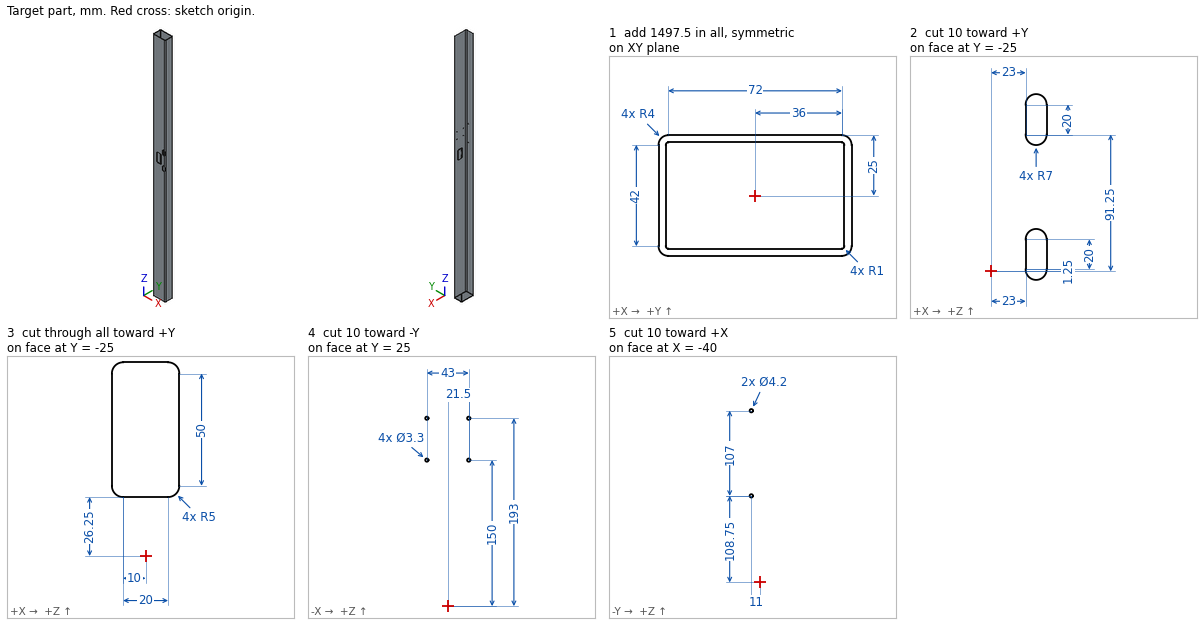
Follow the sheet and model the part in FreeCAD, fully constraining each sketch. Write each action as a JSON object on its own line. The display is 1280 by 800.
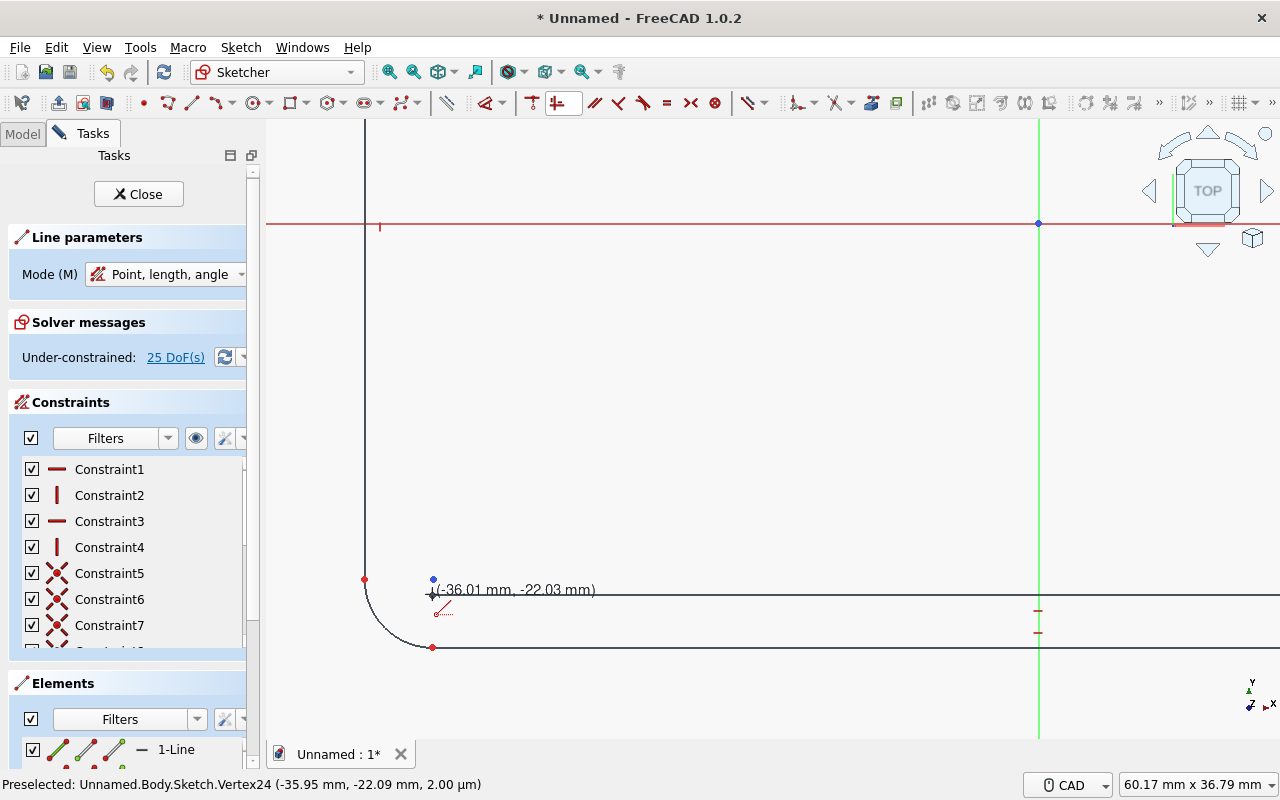
{"action": "left_click", "coordinate": [415, 578]}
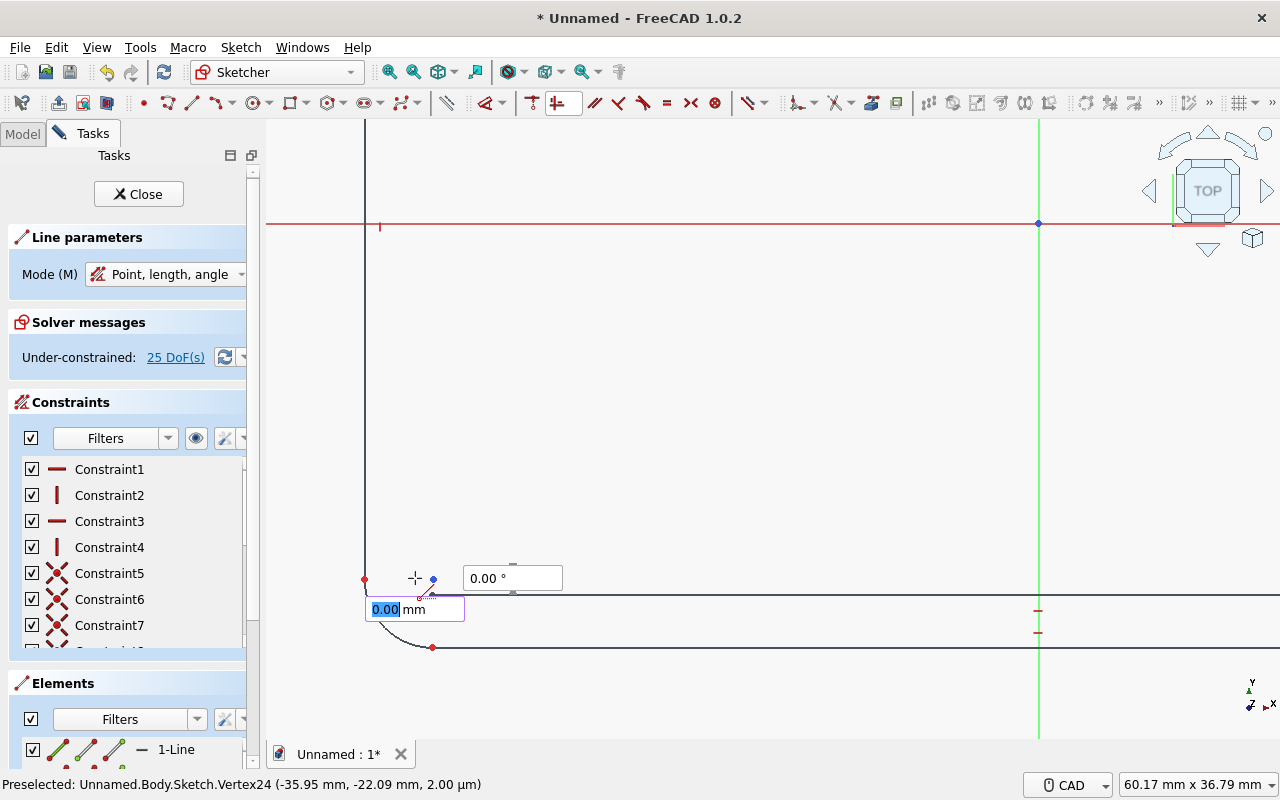
{"action": "scroll", "coordinate": [432, 596], "scroll_direction": "down", "scroll_amount": 4}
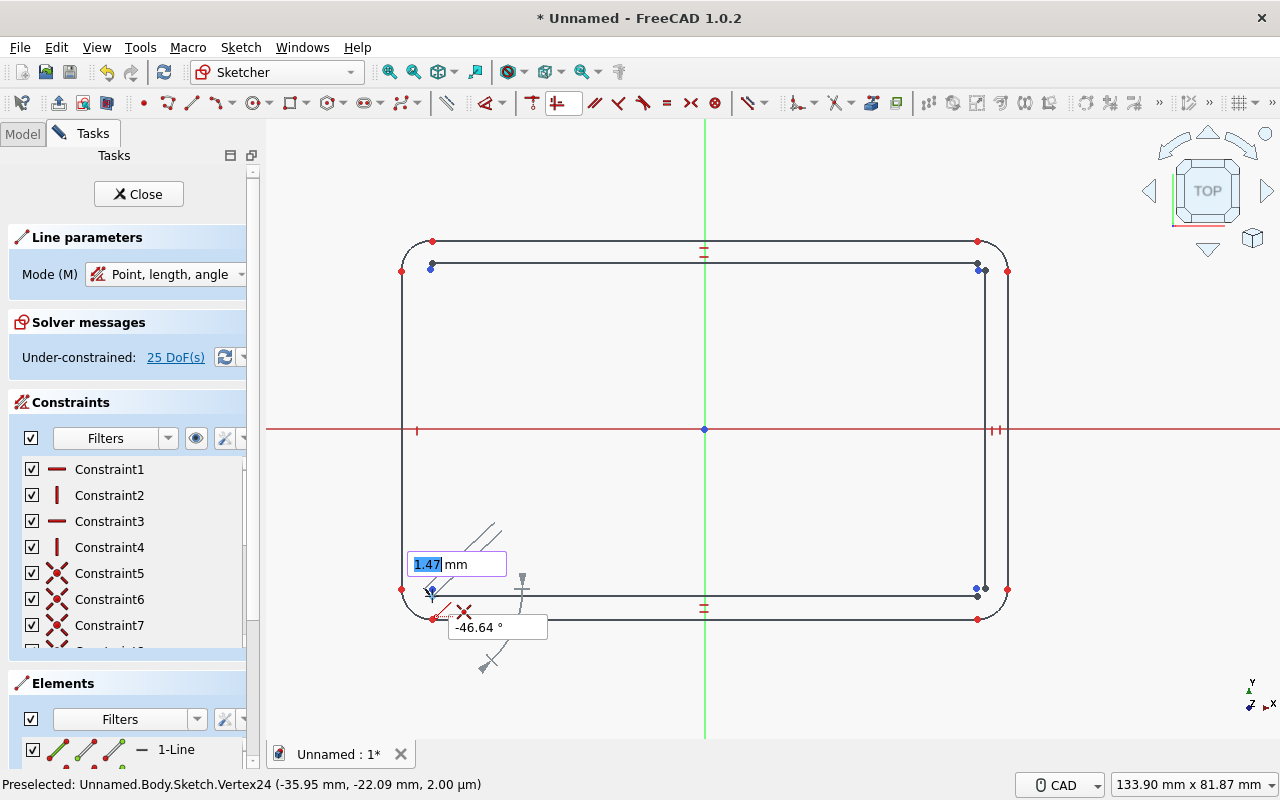
{"action": "scroll", "coordinate": [425, 270], "scroll_direction": "up", "scroll_amount": 4}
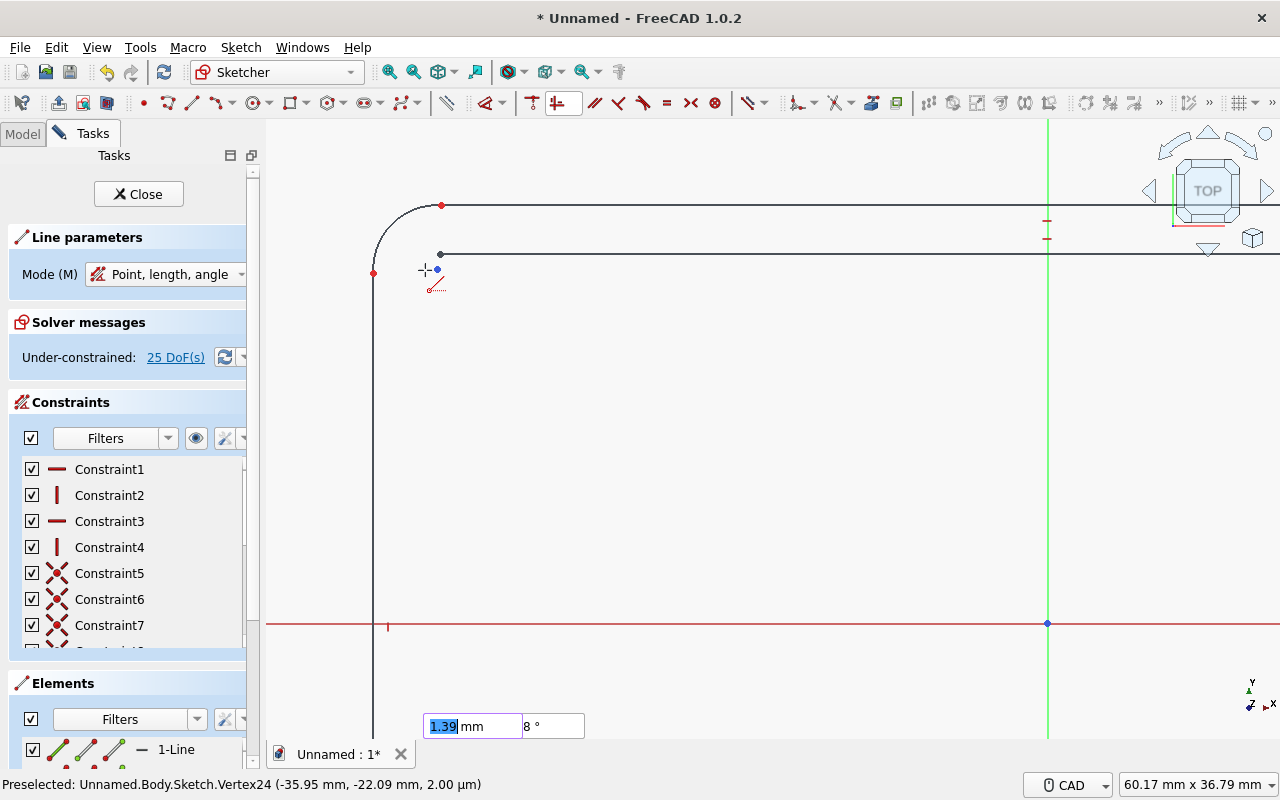
{"action": "left_click", "coordinate": [424, 270]}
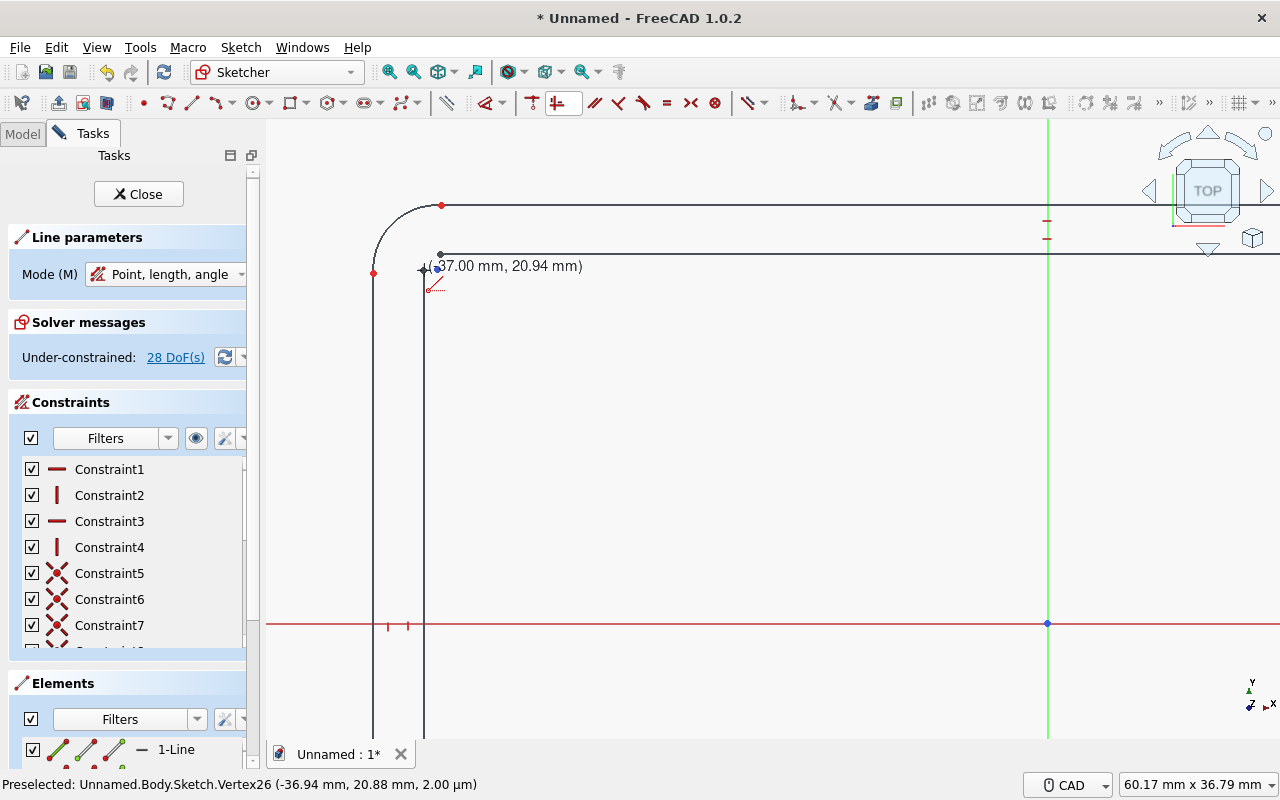
{"action": "left_click", "coordinate": [216, 104]}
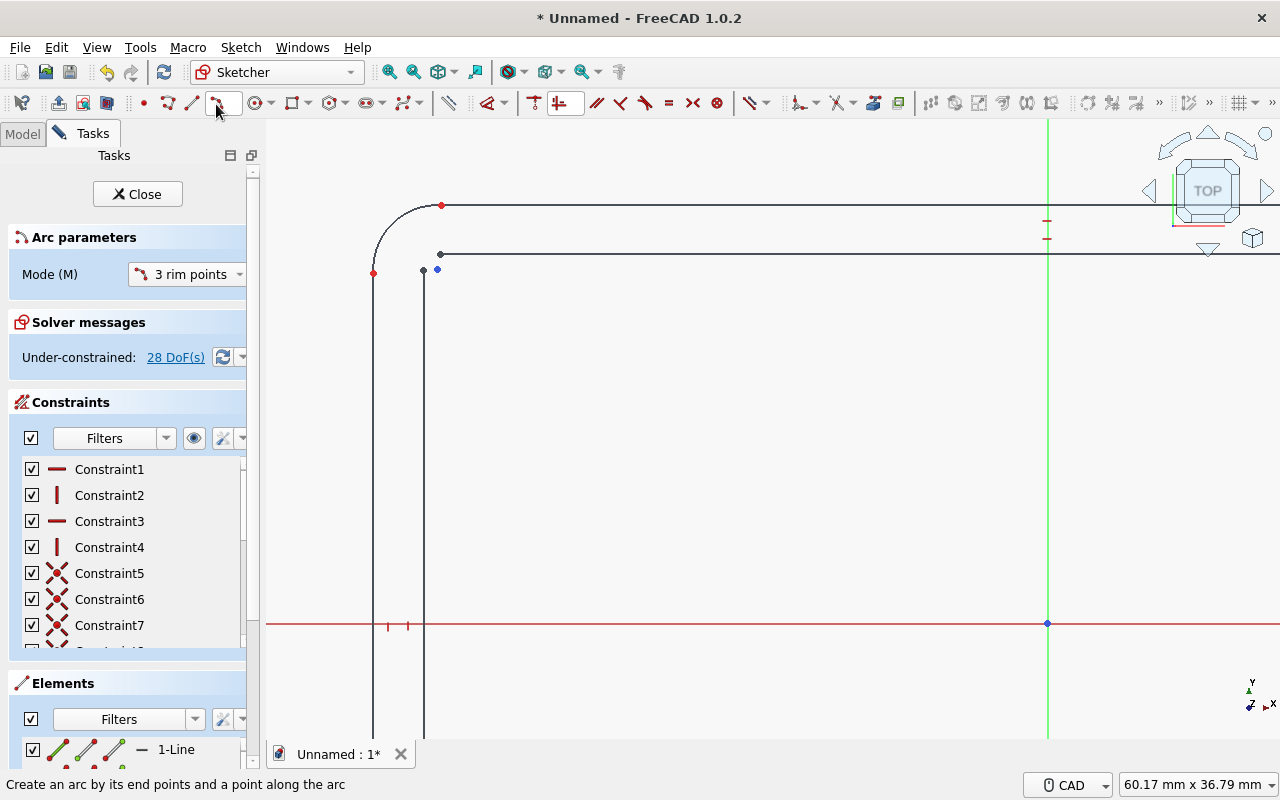
{"action": "scroll", "coordinate": [425, 270], "scroll_direction": "down", "scroll_amount": 4}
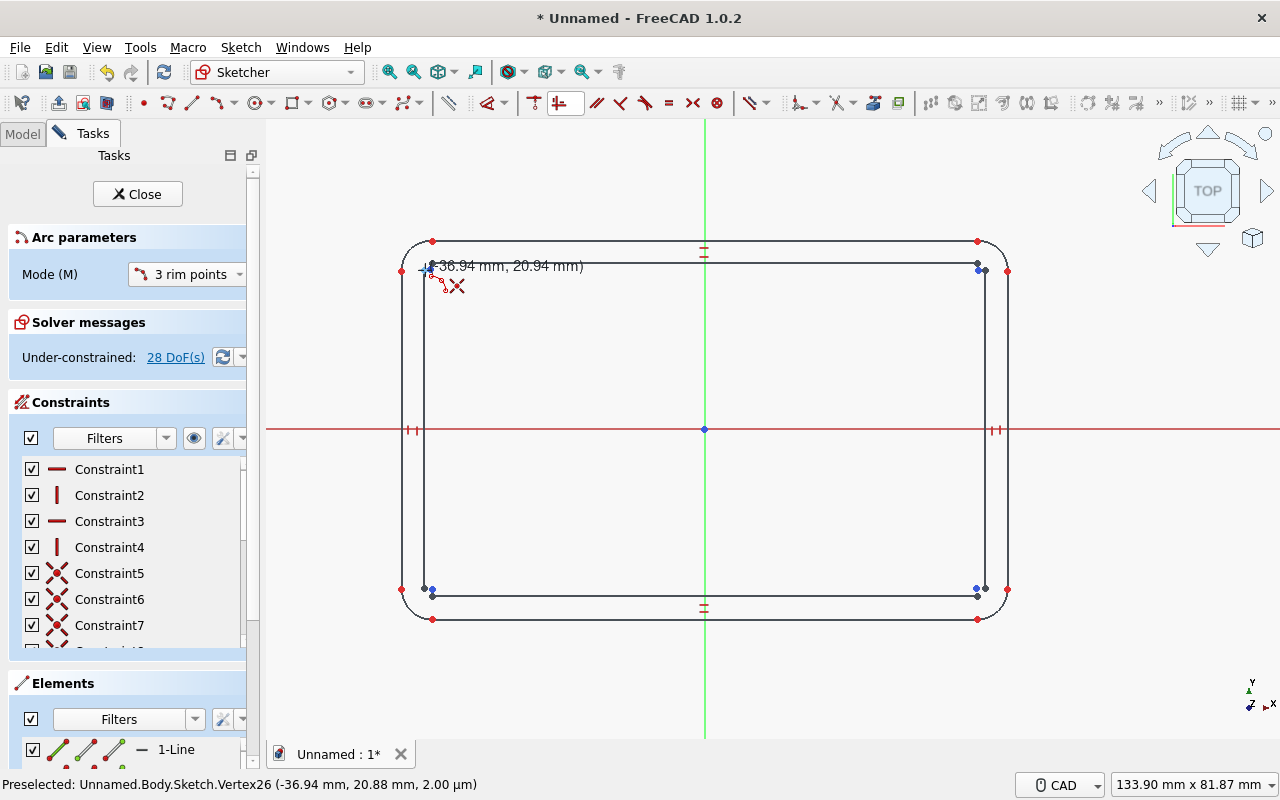
{"action": "scroll", "coordinate": [977, 263], "scroll_direction": "up", "scroll_amount": 4}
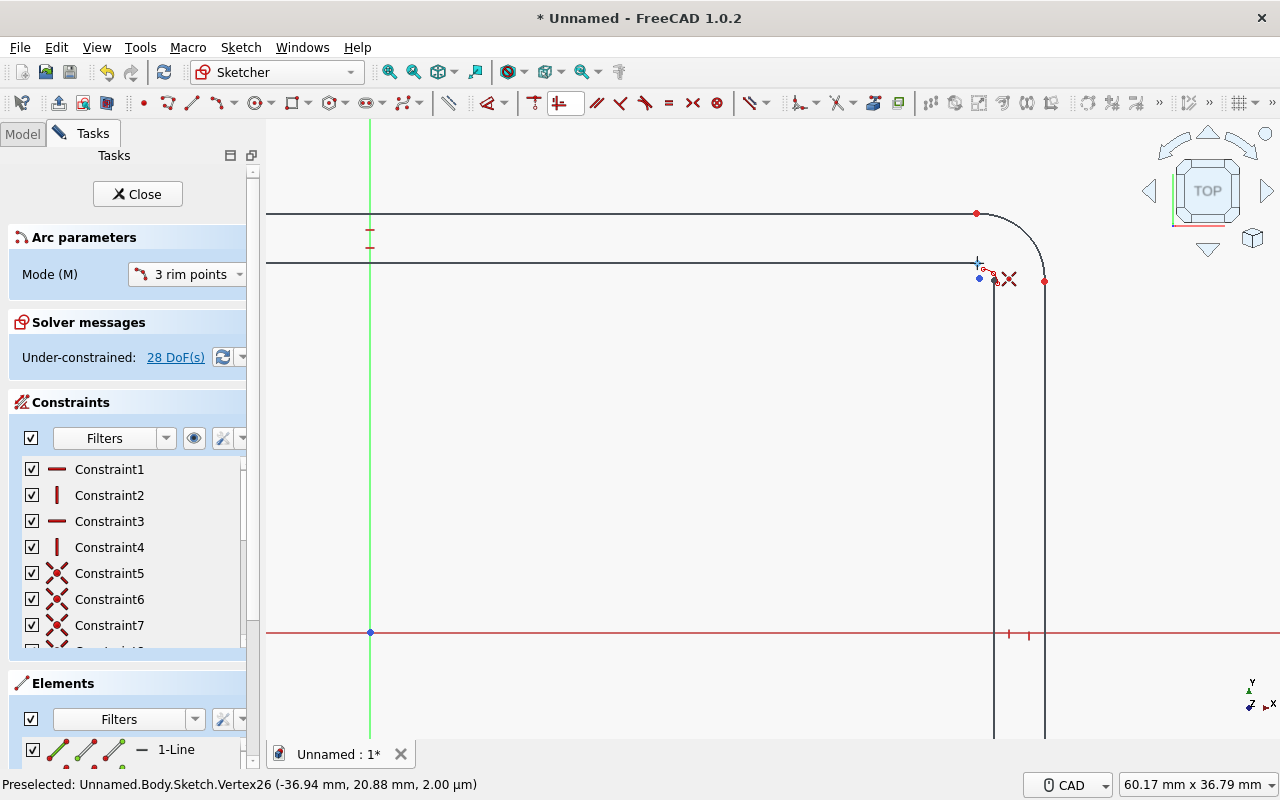
{"action": "left_click", "coordinate": [977, 263]}
{"action": "left_click", "coordinate": [994, 280]}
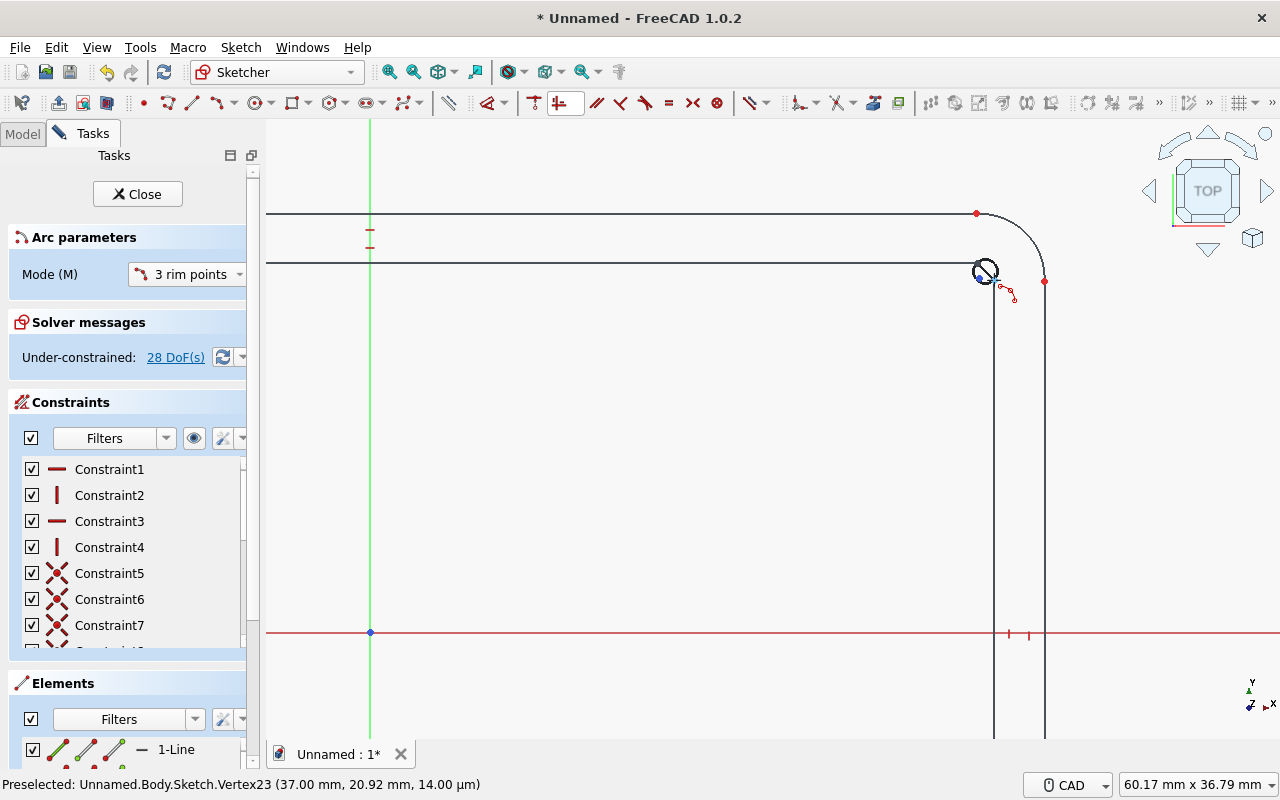
{"action": "scroll", "coordinate": [989, 267], "scroll_direction": "up", "scroll_amount": 6}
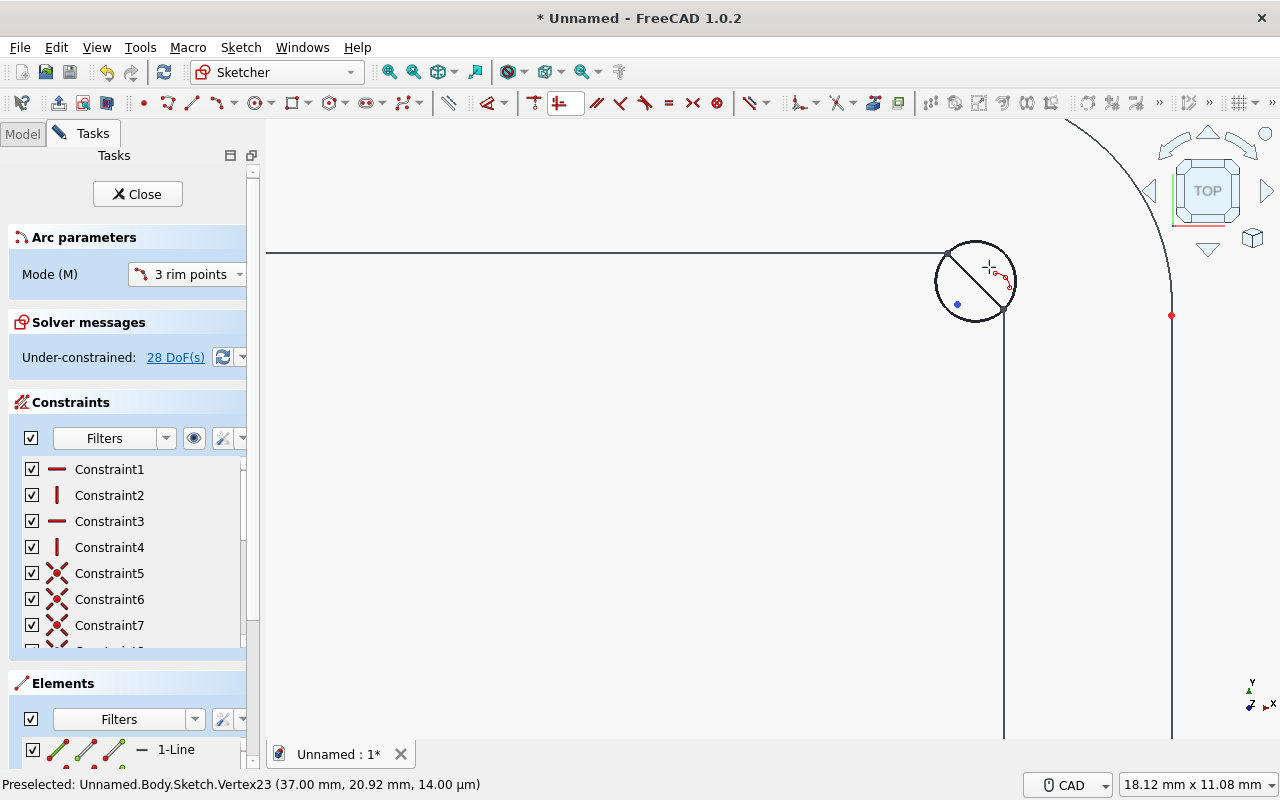
{"action": "left_click", "coordinate": [987, 265]}